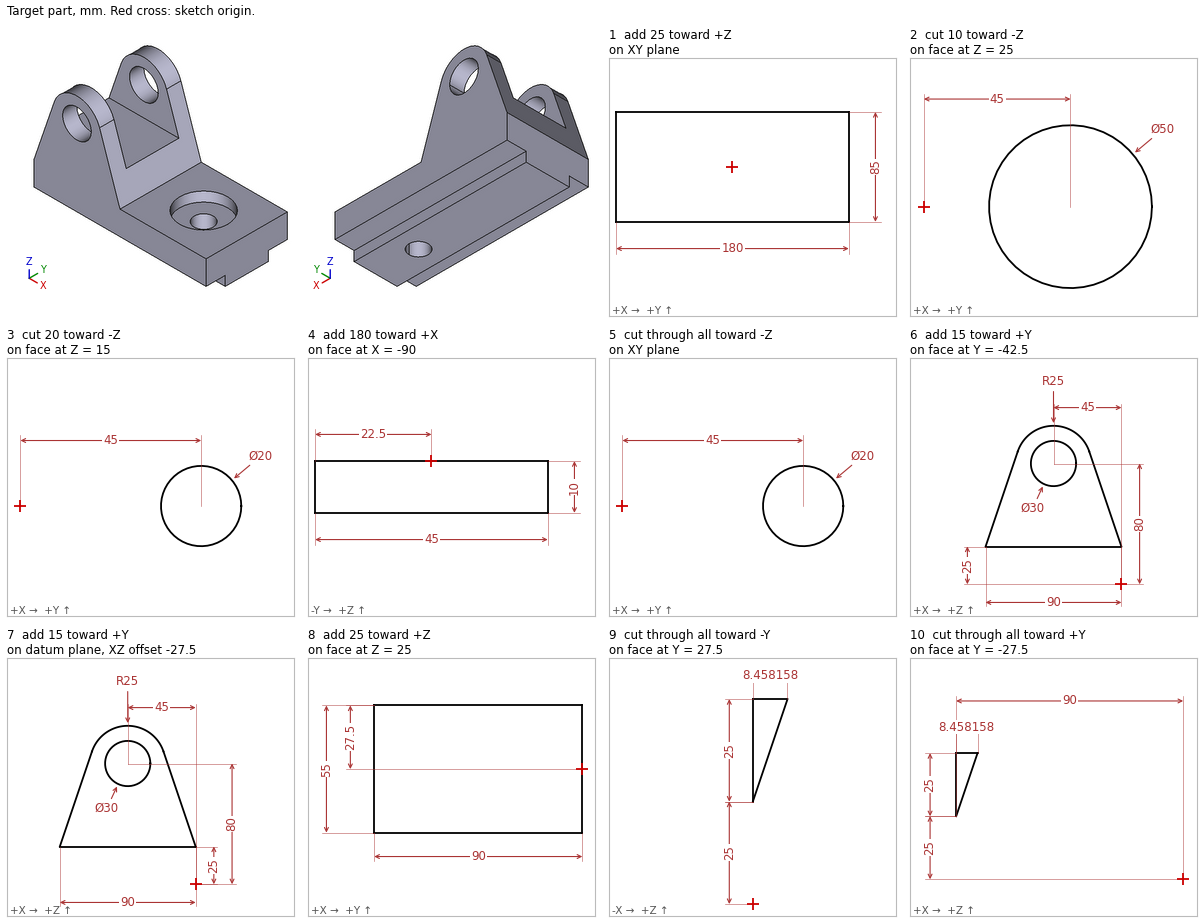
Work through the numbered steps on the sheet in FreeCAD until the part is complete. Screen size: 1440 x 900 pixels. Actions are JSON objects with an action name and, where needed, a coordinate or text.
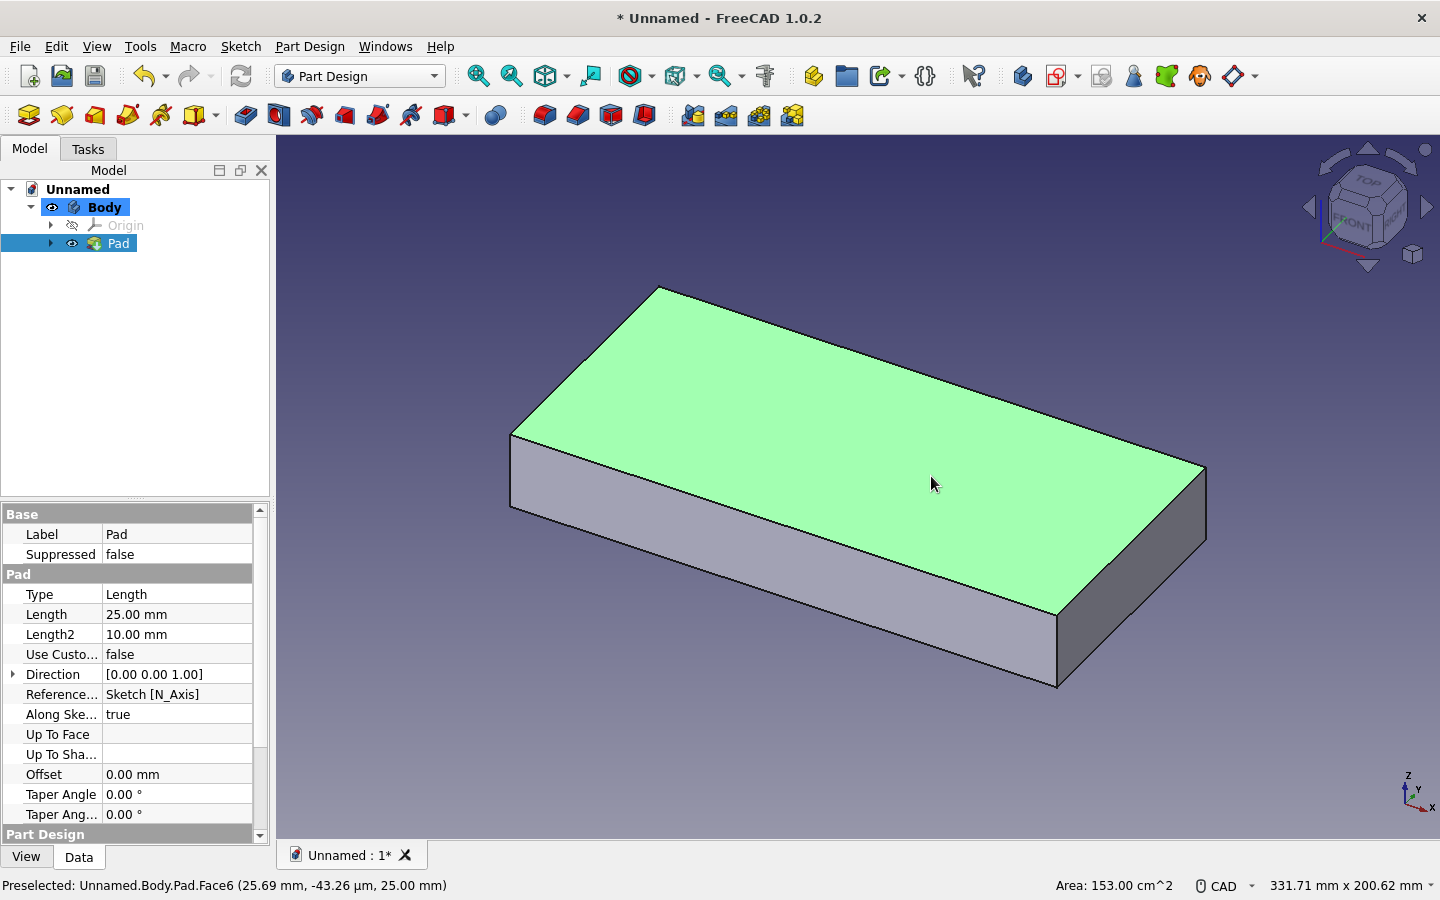
{"action": "left_click", "coordinate": [1056, 76]}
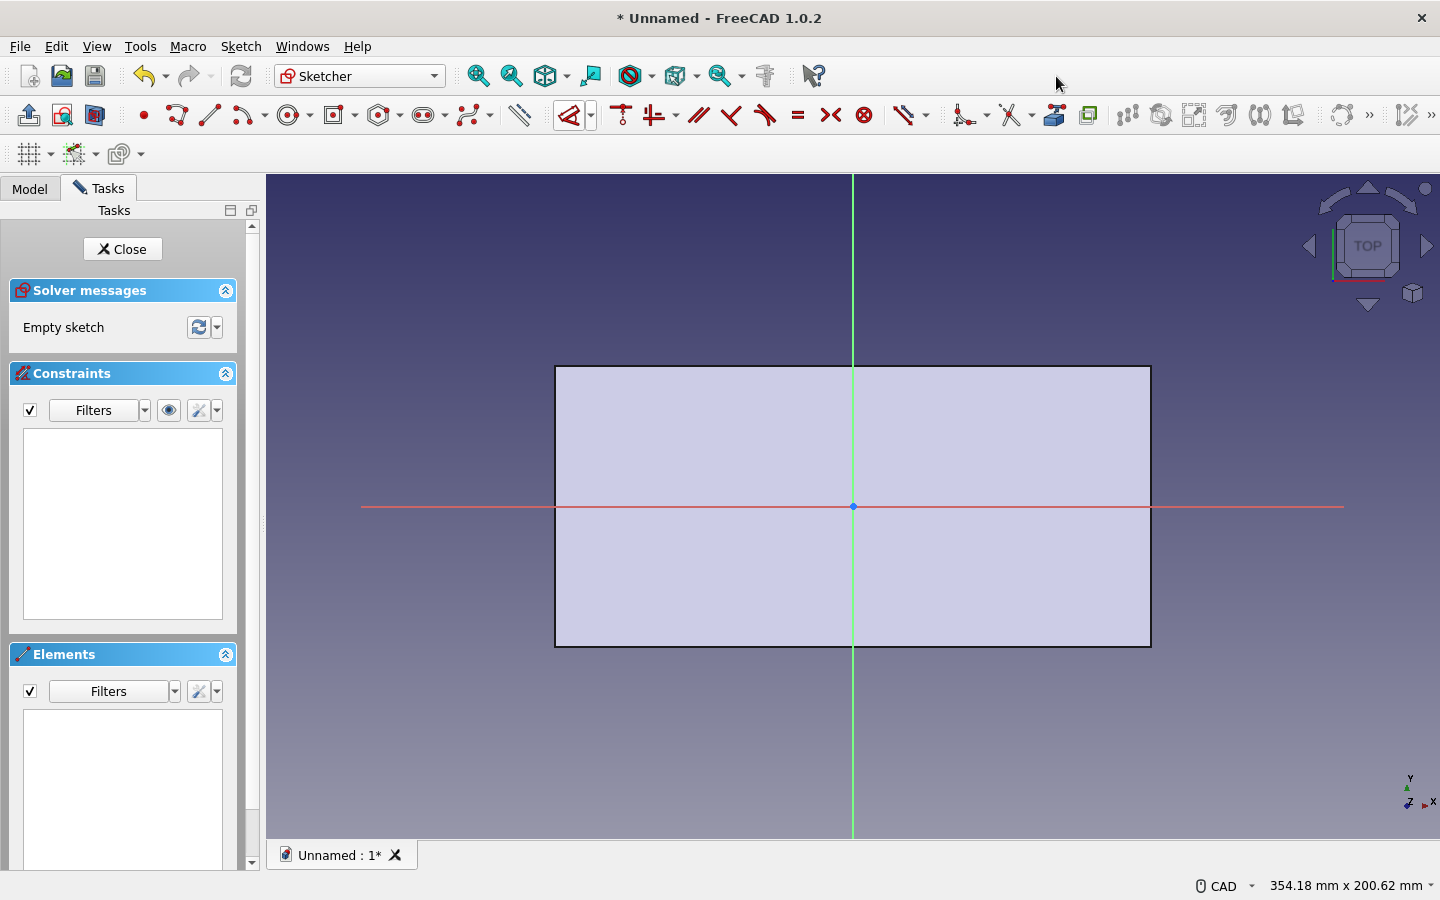
{"action": "scroll", "coordinate": [1076, 507], "scroll_direction": "up", "scroll_amount": 5}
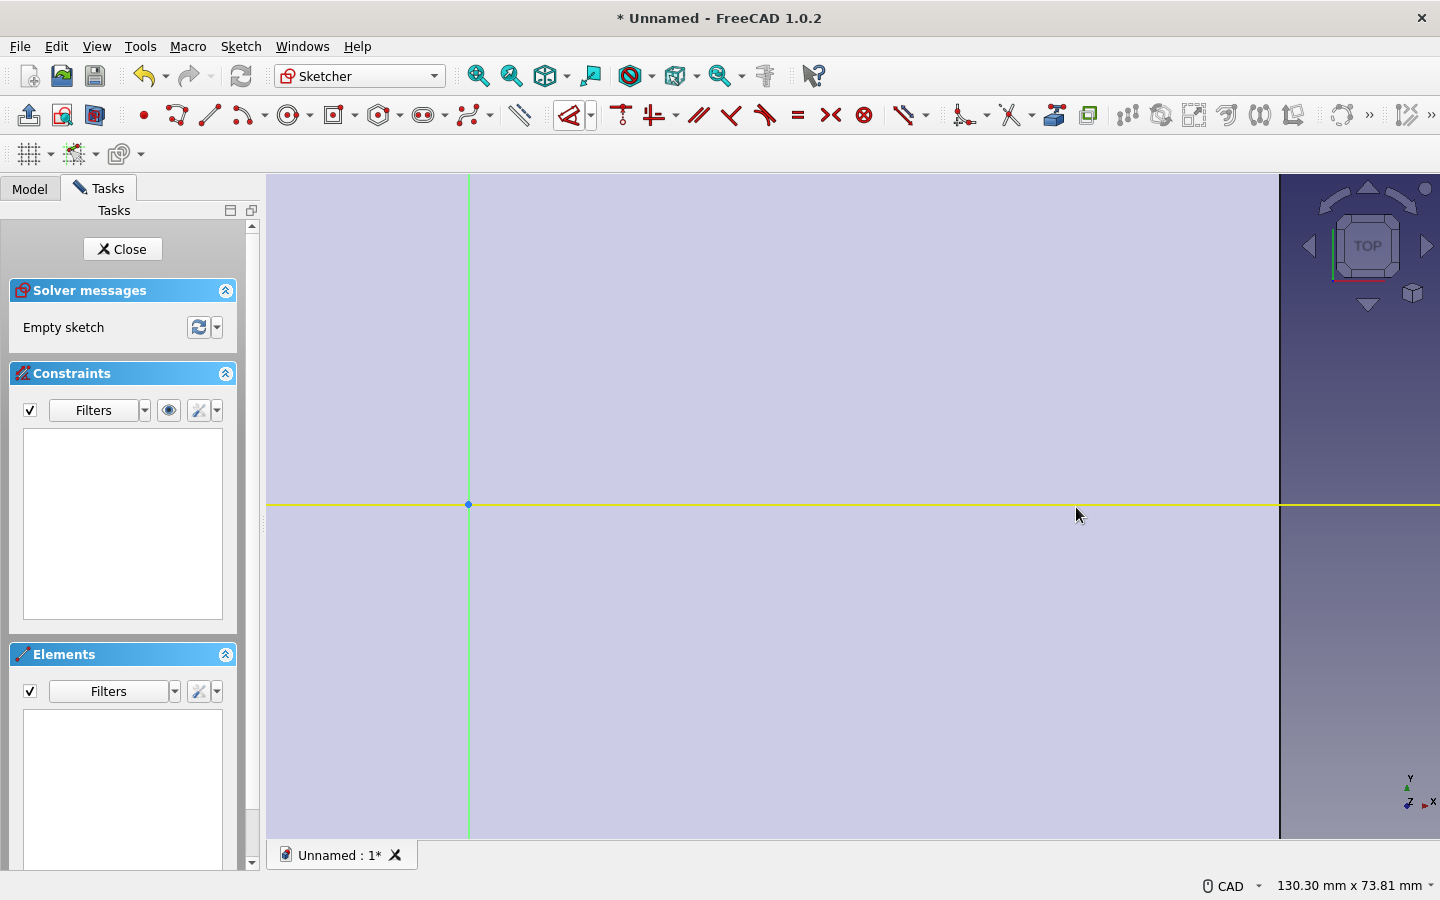
{"action": "left_click", "coordinate": [288, 116]}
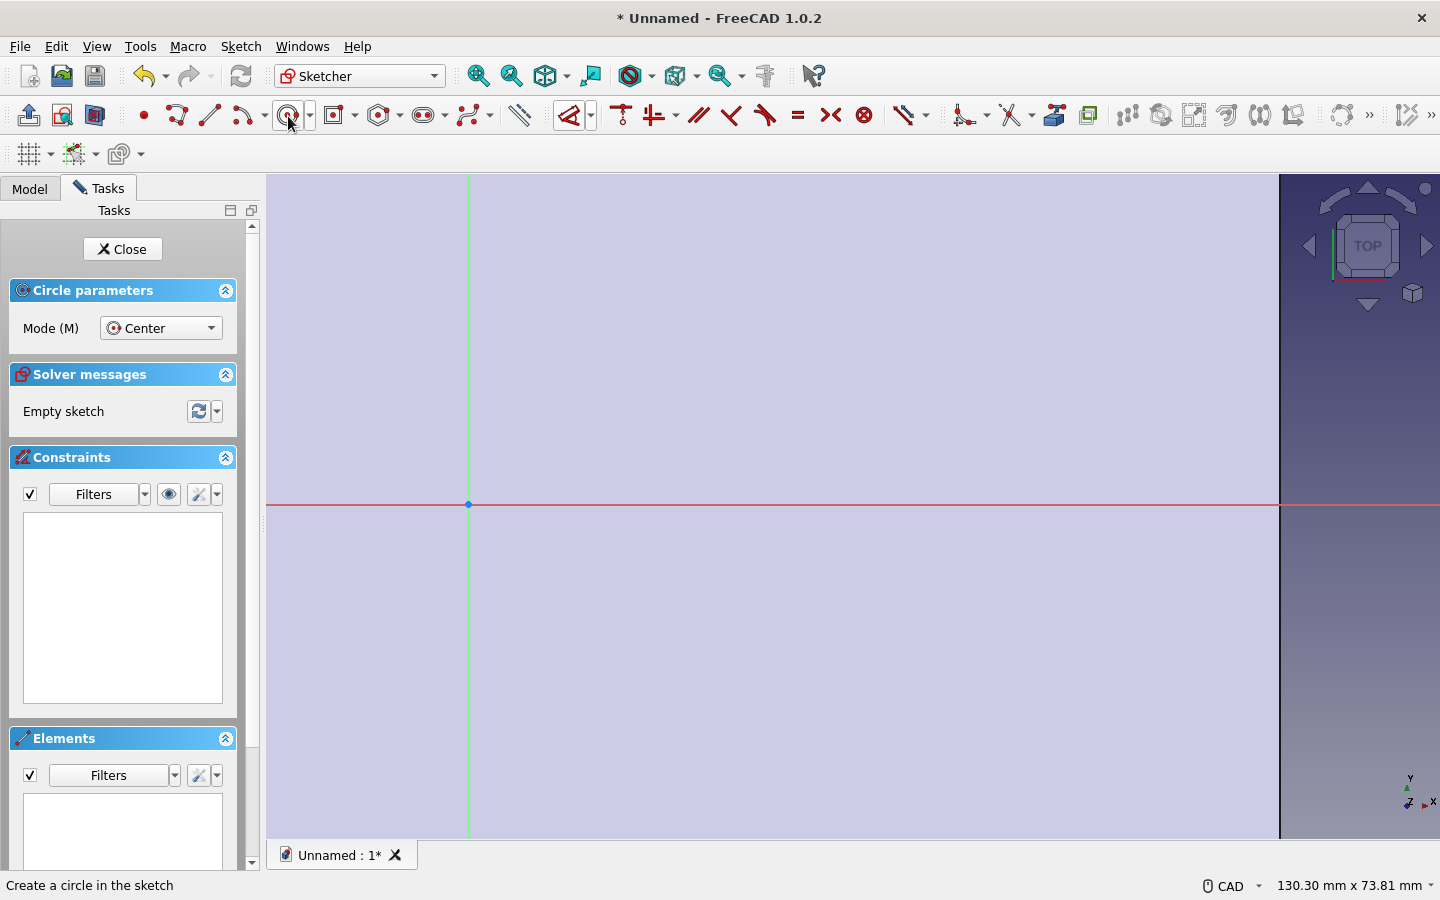
{"action": "left_click", "coordinate": [874, 505]}
{"action": "mouse_move", "coordinate": [1033, 346]}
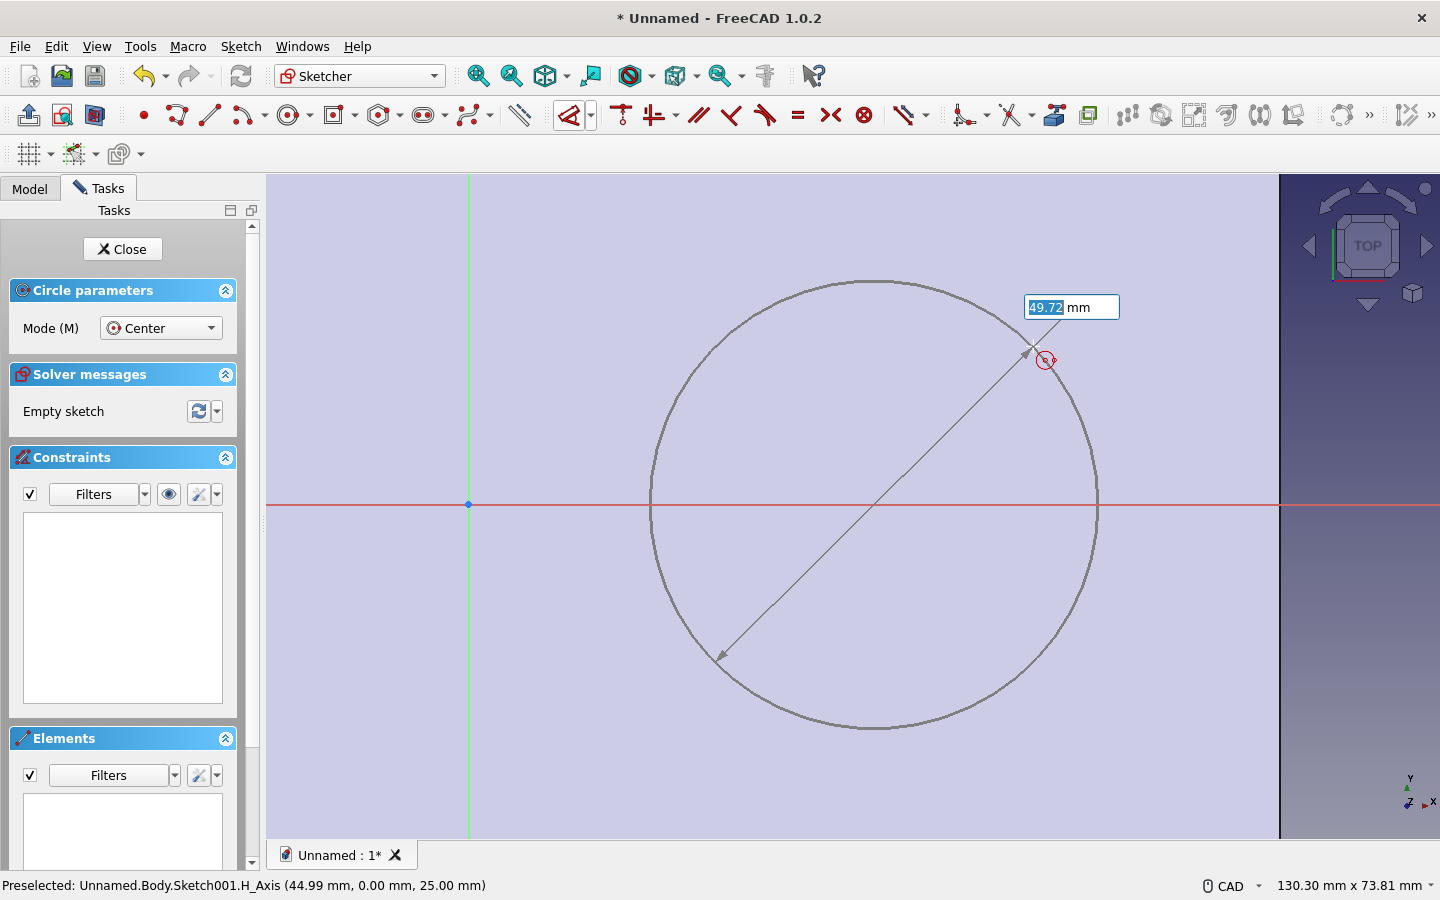
{"action": "type", "text": "50"}
{"action": "key", "text": "Return"}
{"action": "key", "text": "Escape"}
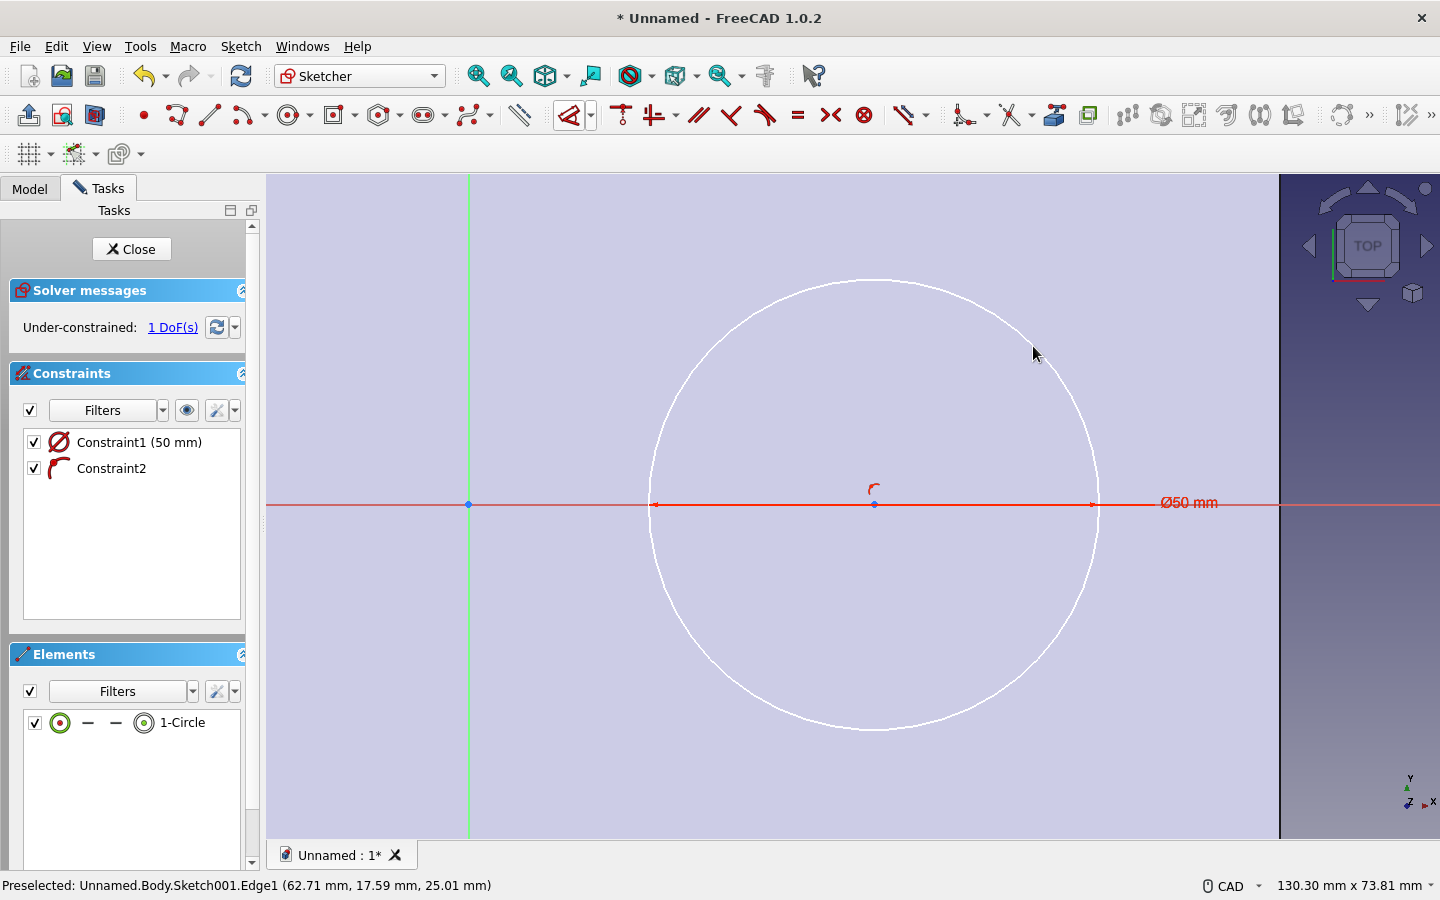
{"action": "left_click", "coordinate": [568, 116]}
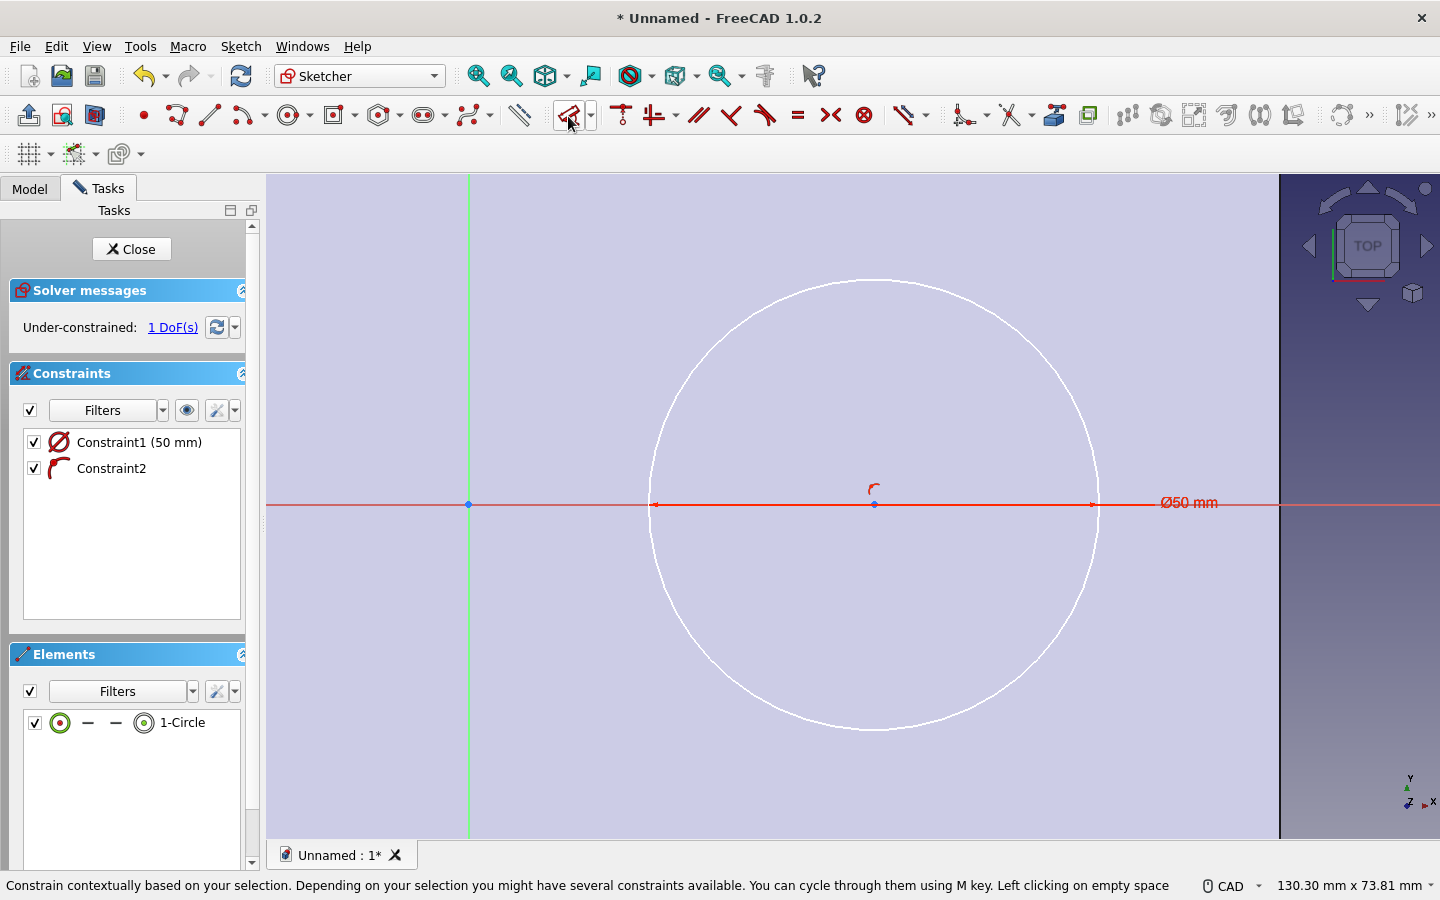
{"action": "left_click", "coordinate": [874, 505]}
{"action": "left_click", "coordinate": [671, 539]}